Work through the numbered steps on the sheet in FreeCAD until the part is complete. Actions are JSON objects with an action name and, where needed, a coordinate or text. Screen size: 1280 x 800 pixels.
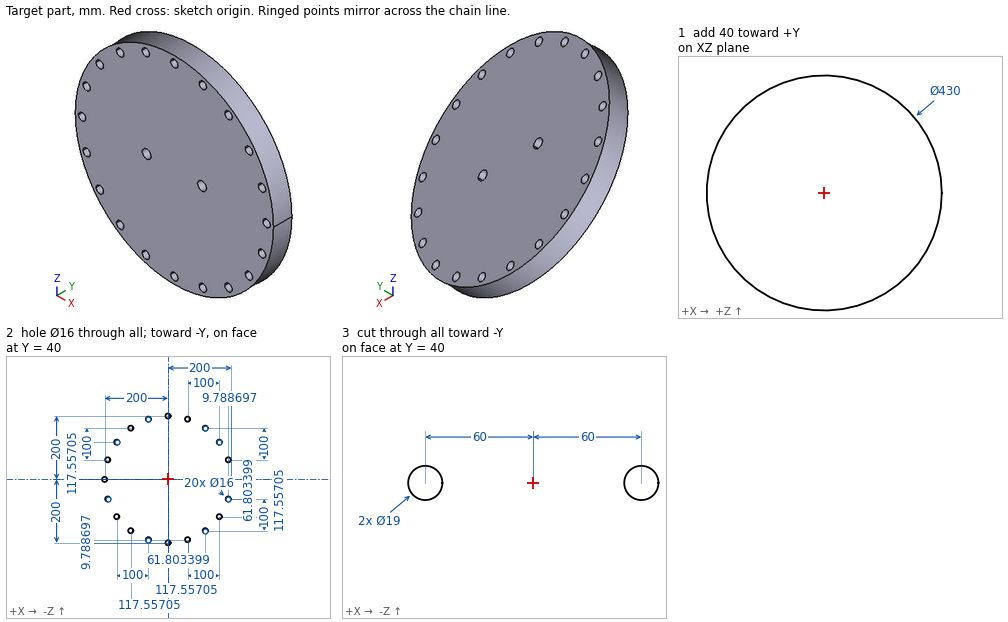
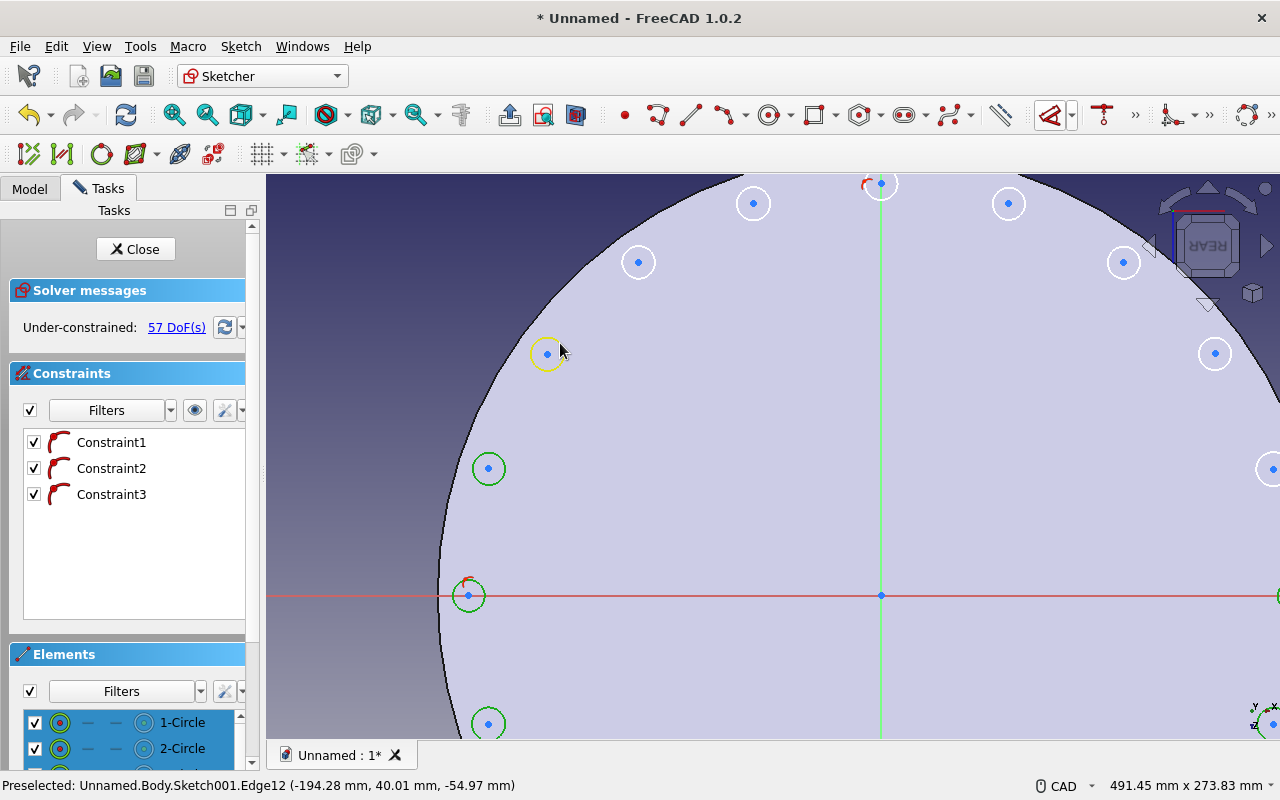
{"action": "left_click", "coordinate": [559, 342]}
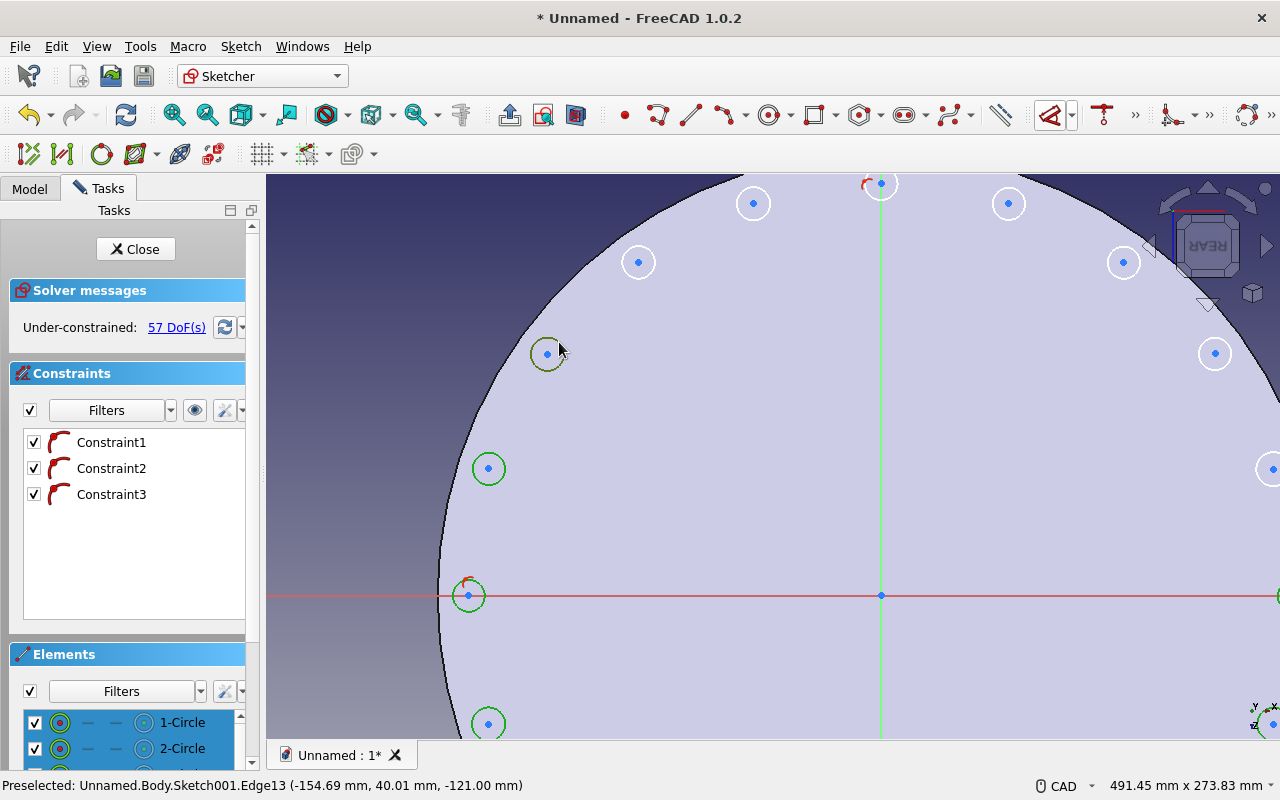
{"action": "left_click", "coordinate": [650, 251]}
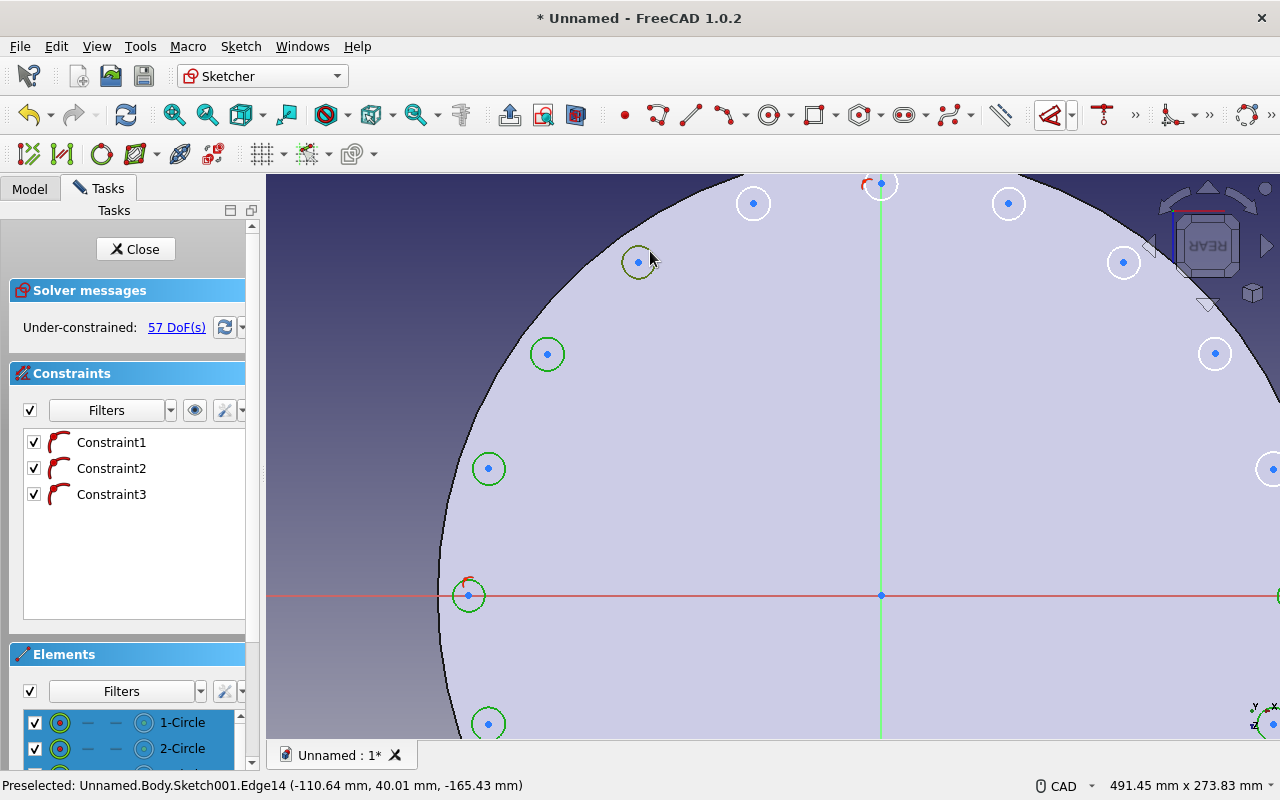
{"action": "left_click", "coordinate": [742, 216]}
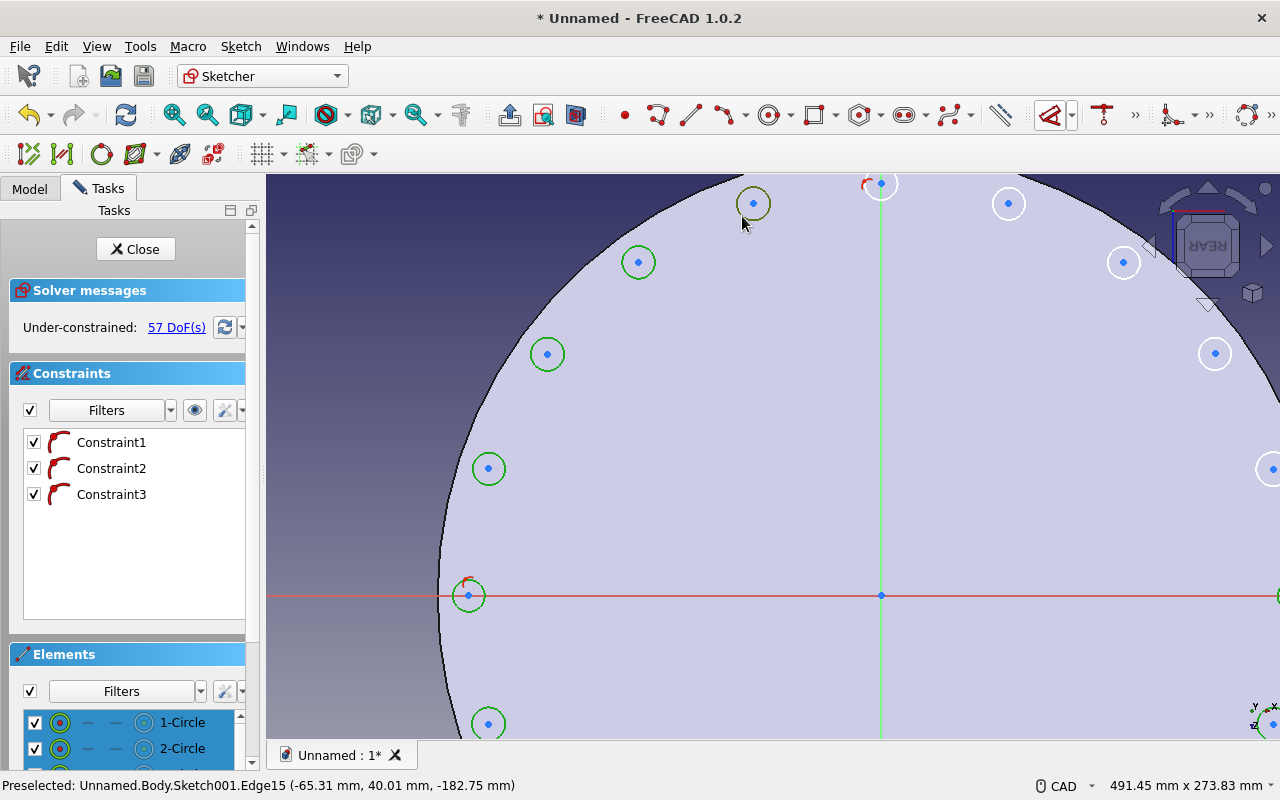
{"action": "scroll", "coordinate": [560, 343], "scroll_direction": "down", "scroll_amount": 4}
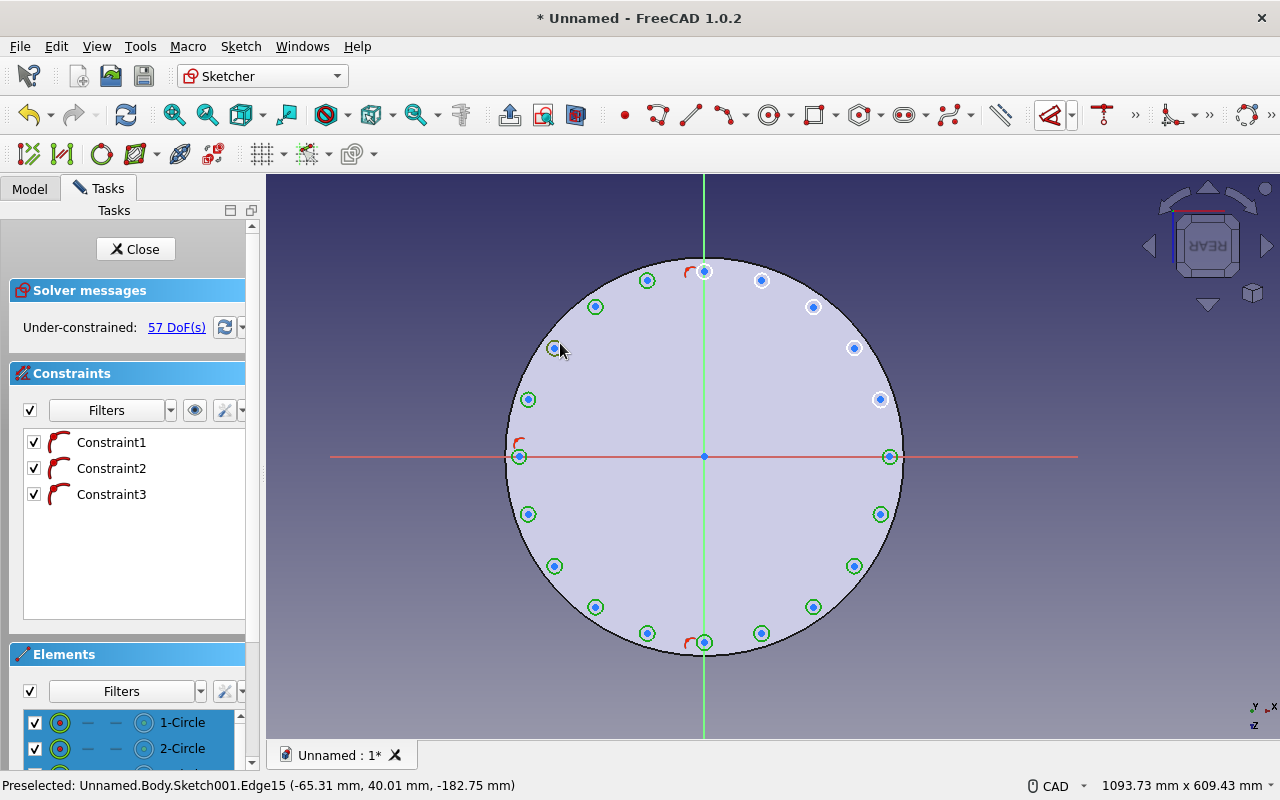
{"action": "scroll", "coordinate": [710, 266], "scroll_direction": "up", "scroll_amount": 5}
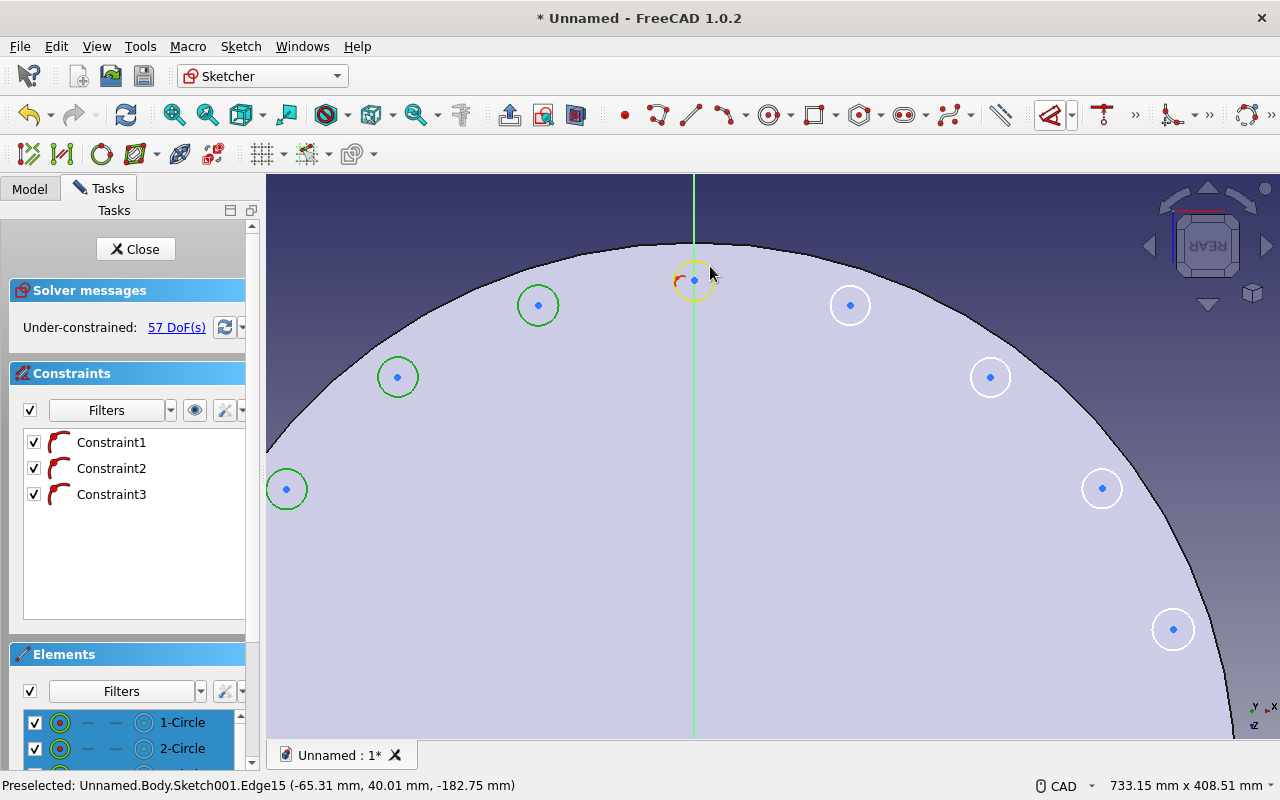
{"action": "left_click", "coordinate": [708, 267]}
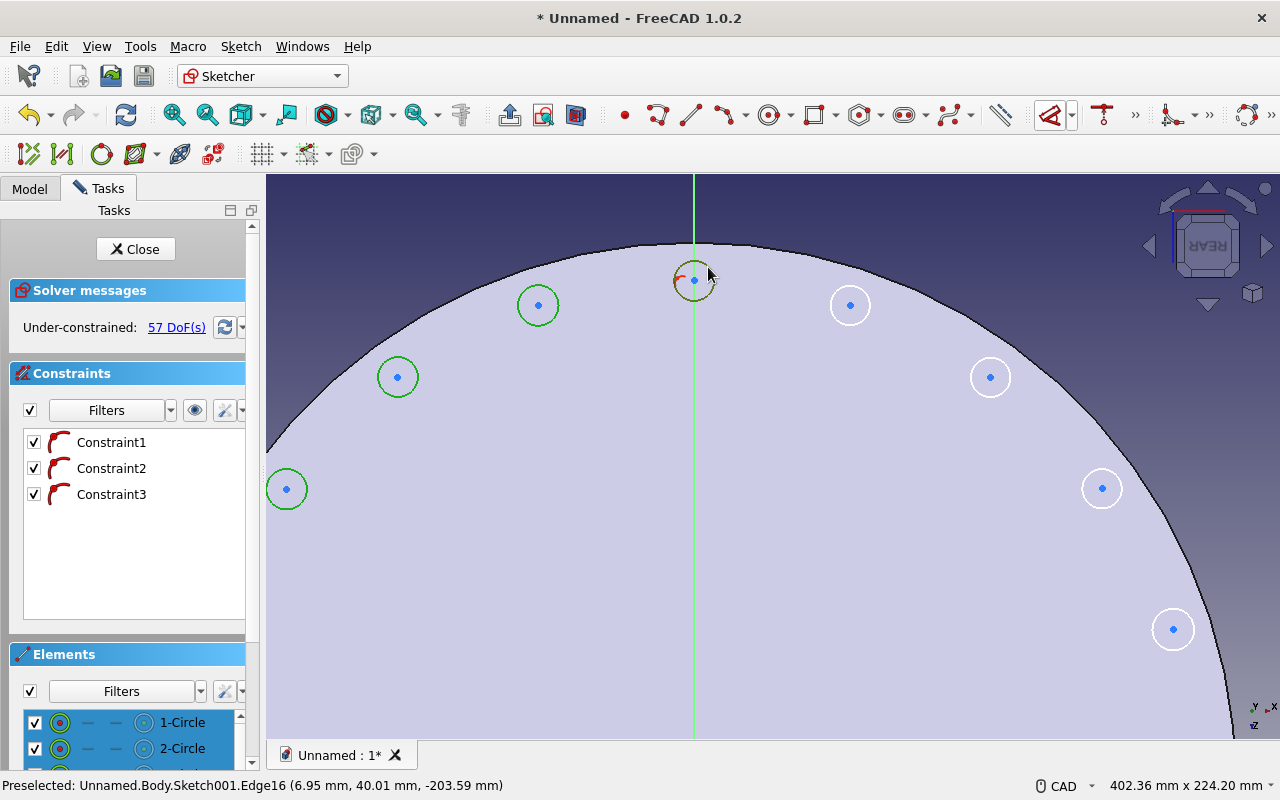
{"action": "left_click", "coordinate": [864, 292]}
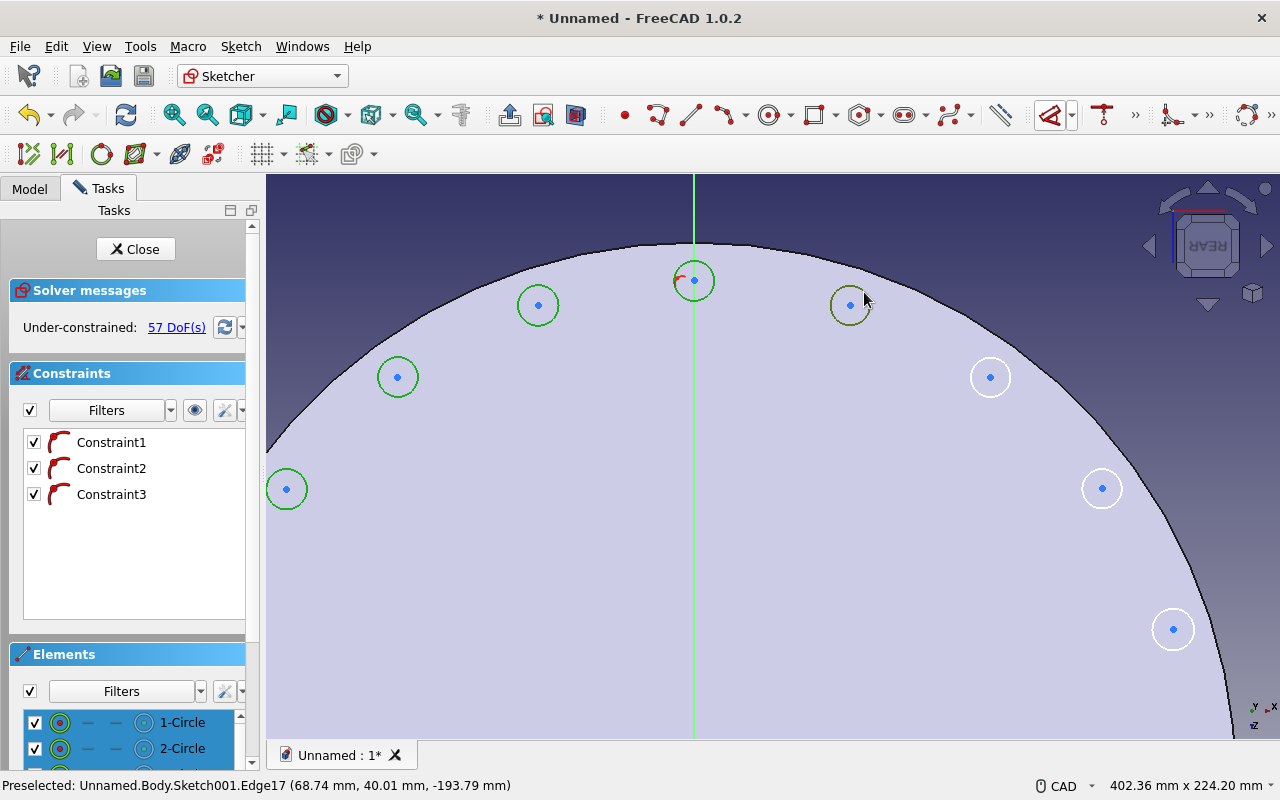
{"action": "left_click", "coordinate": [1005, 363]}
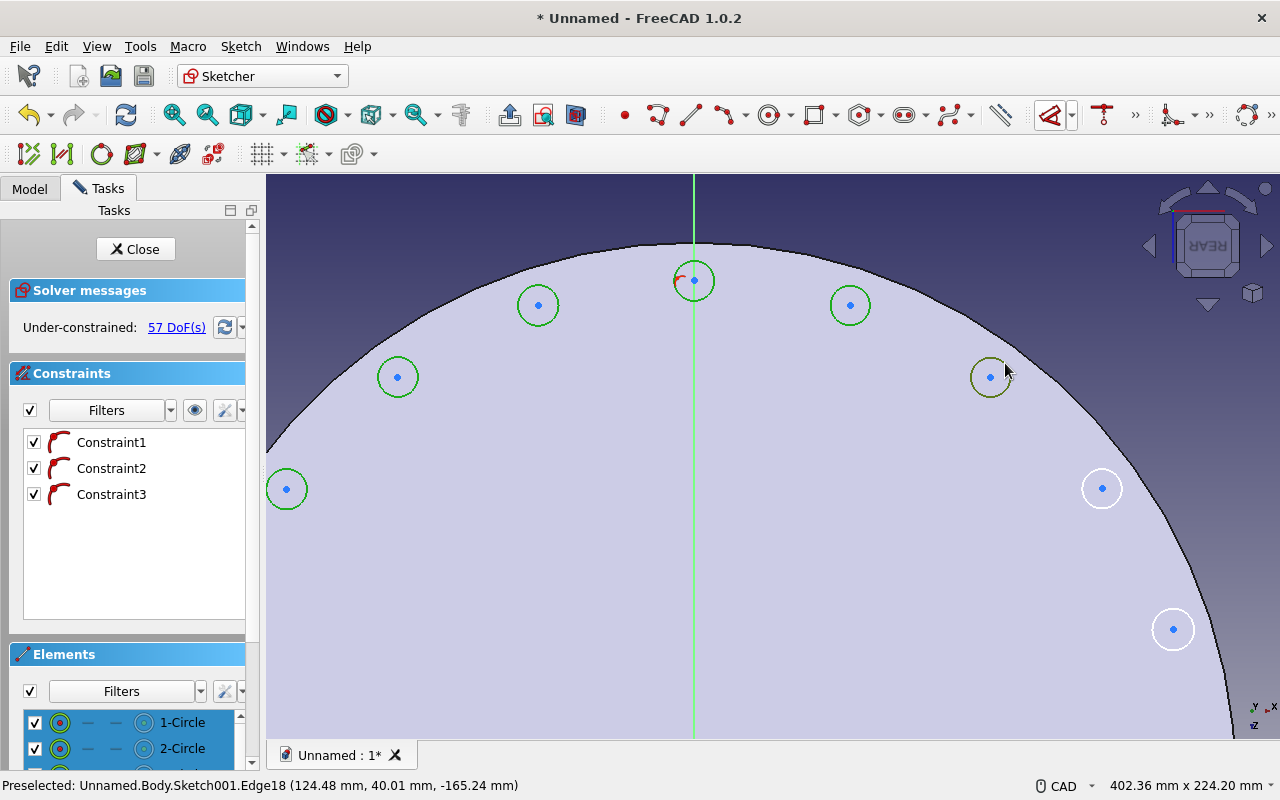
{"action": "left_click", "coordinate": [1088, 475]}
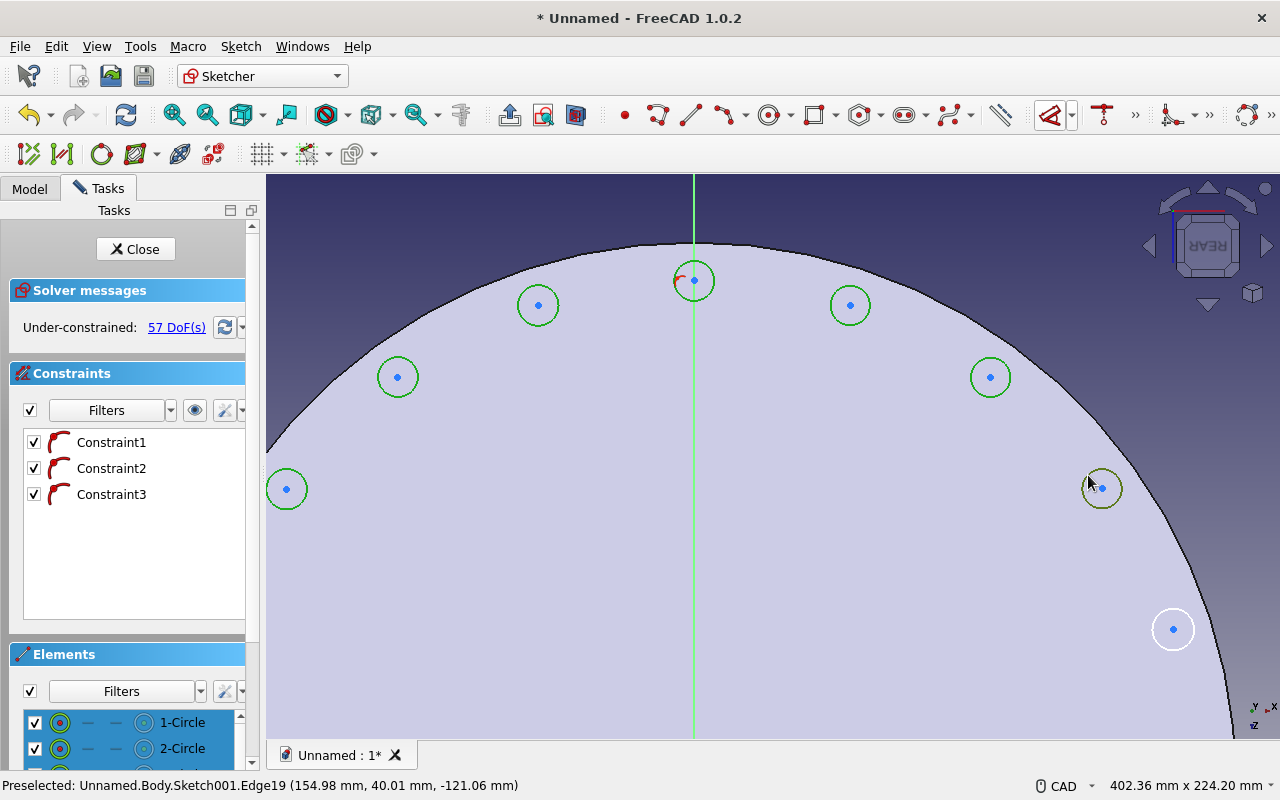
{"action": "scroll", "coordinate": [710, 266], "scroll_direction": "down", "scroll_amount": 5}